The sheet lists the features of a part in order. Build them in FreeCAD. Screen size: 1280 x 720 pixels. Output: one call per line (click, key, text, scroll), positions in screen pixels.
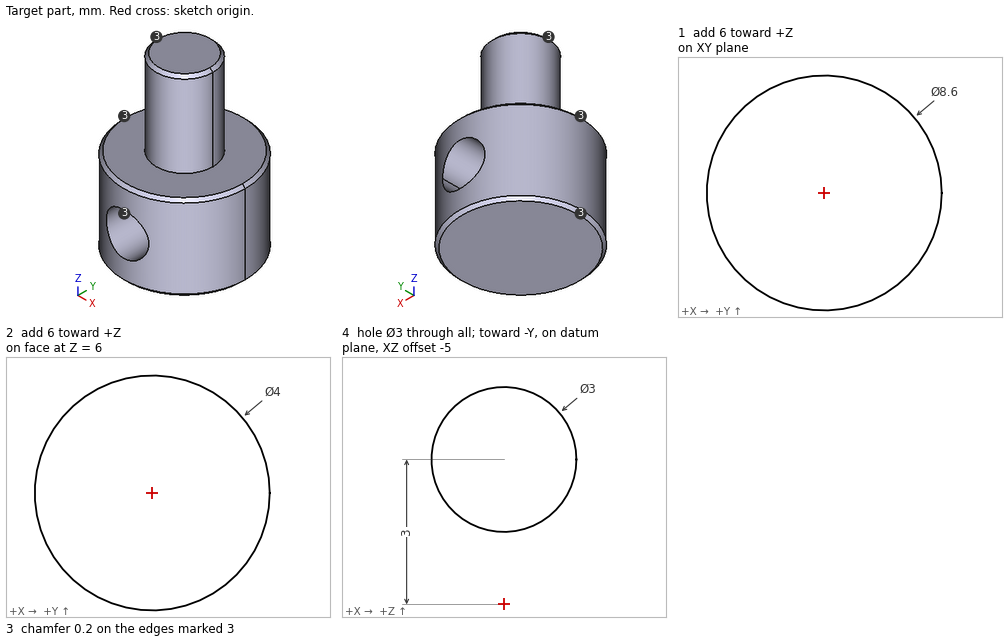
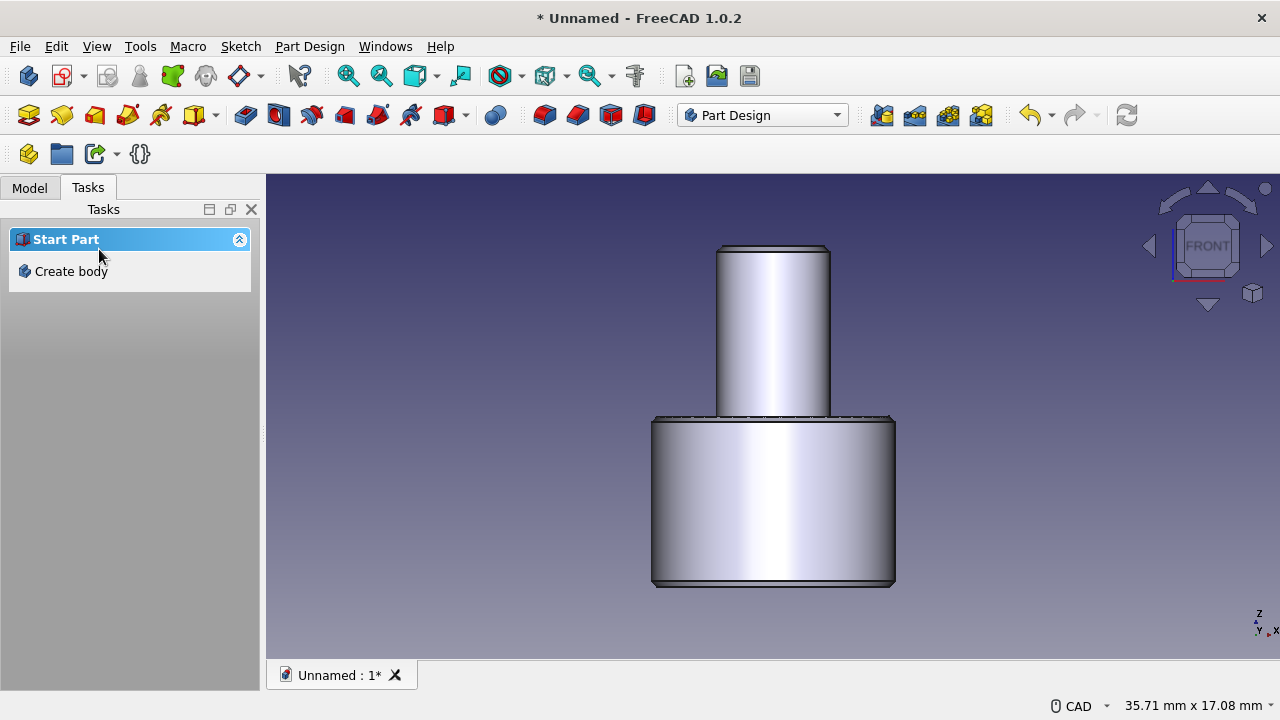
click(30, 188)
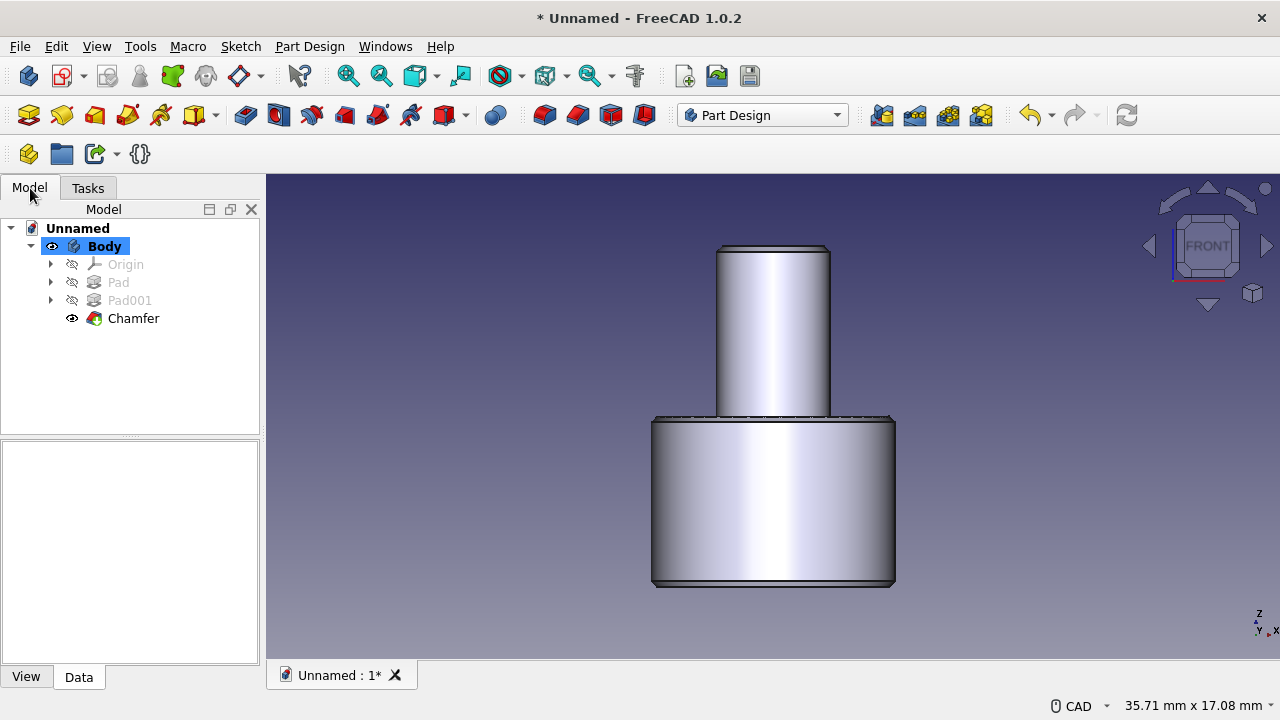
click(51, 264)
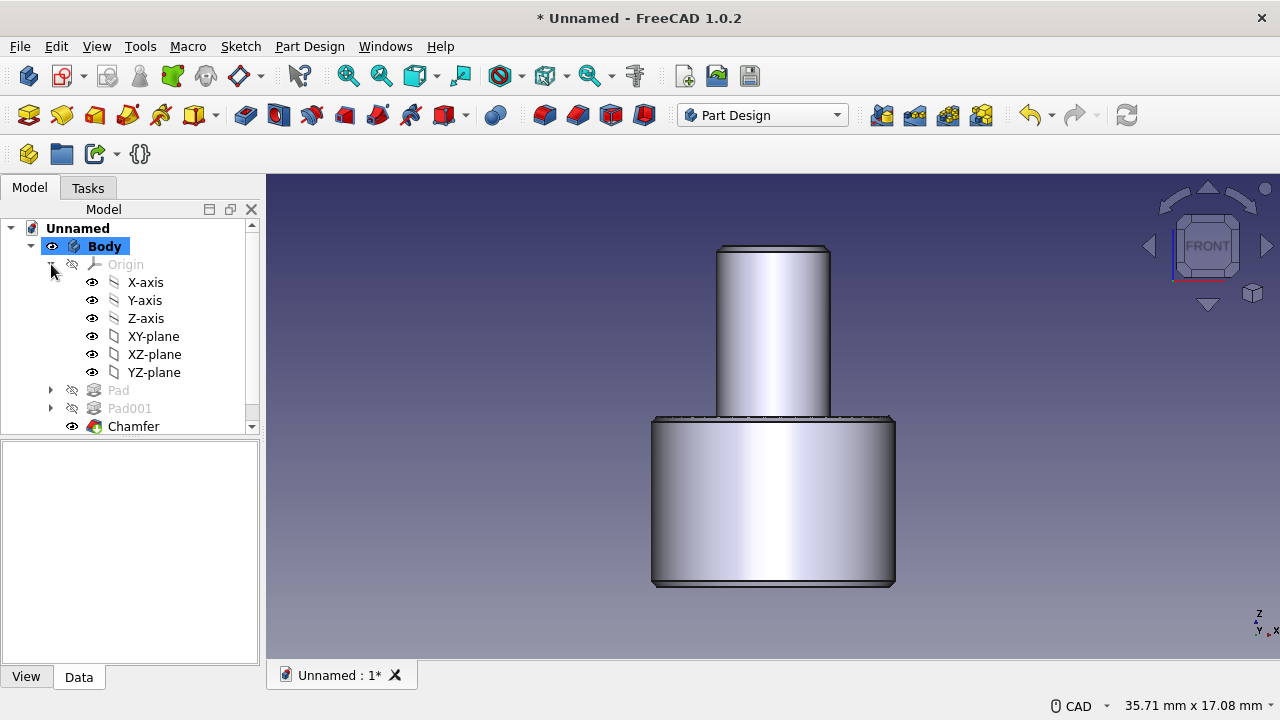
click(137, 354)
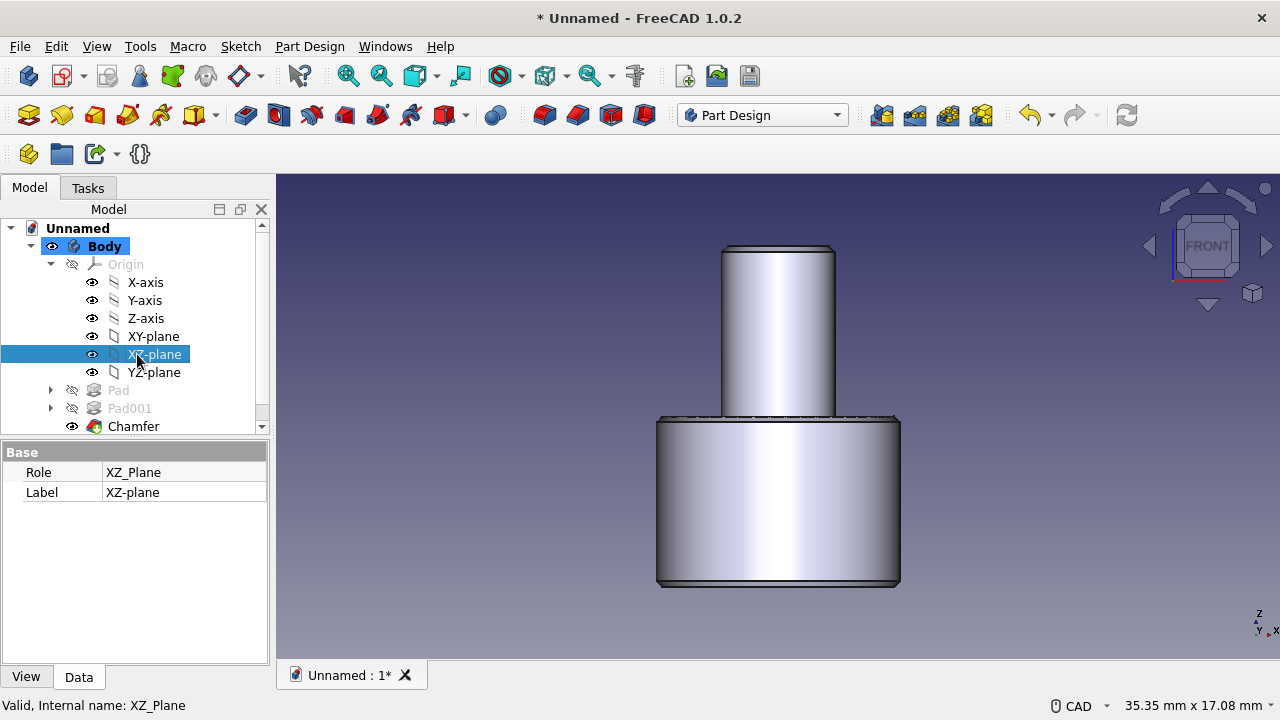
click(238, 76)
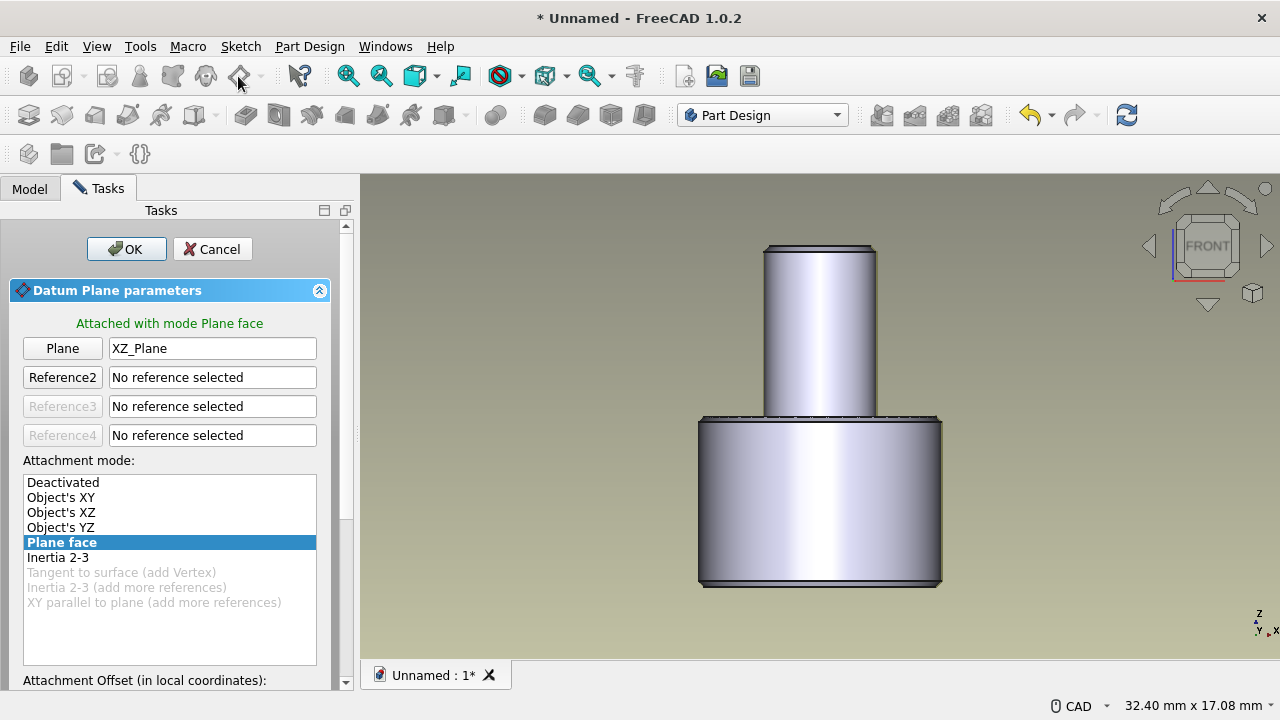
scroll(346, 455, down, 3)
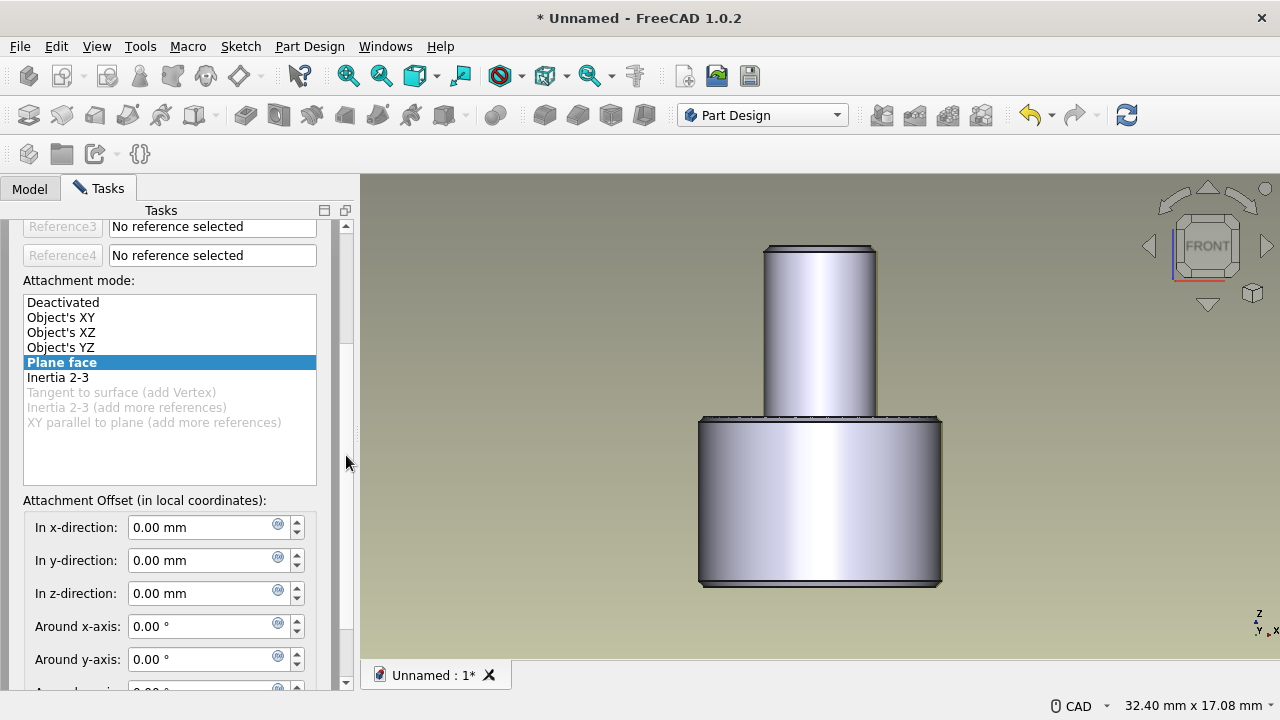
triple_click(210, 594)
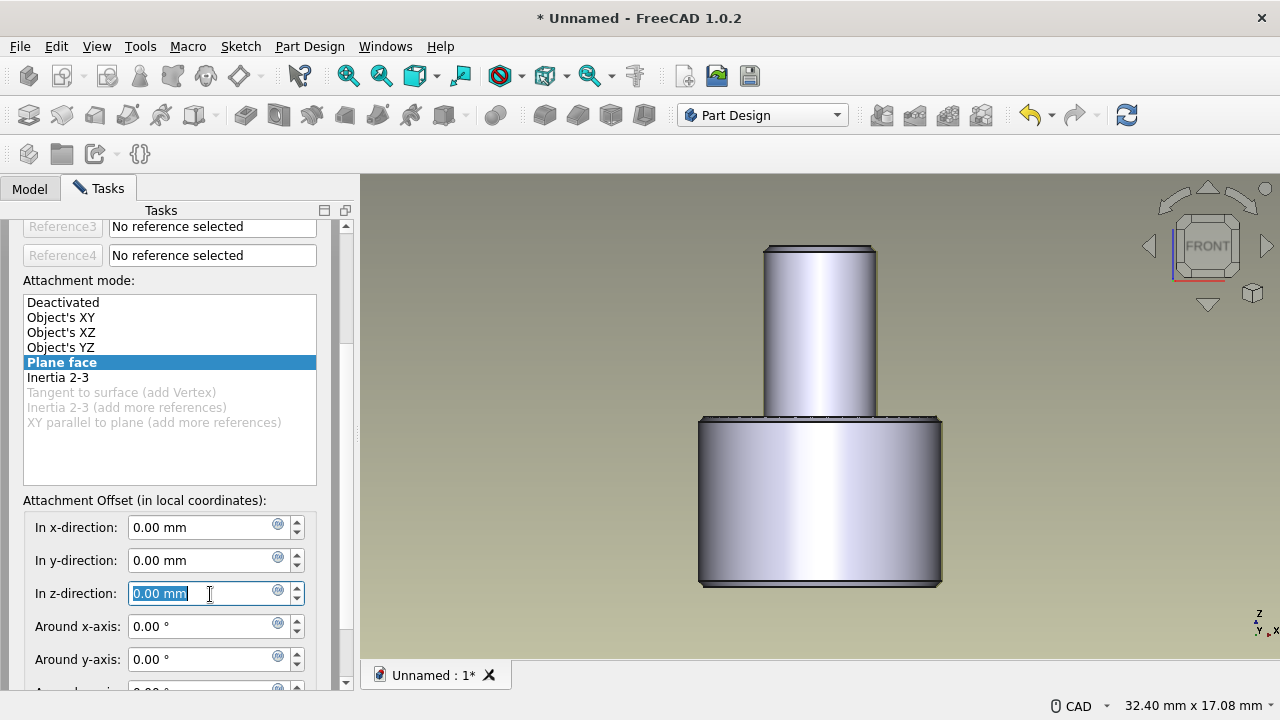
text(-5)
key(Tab)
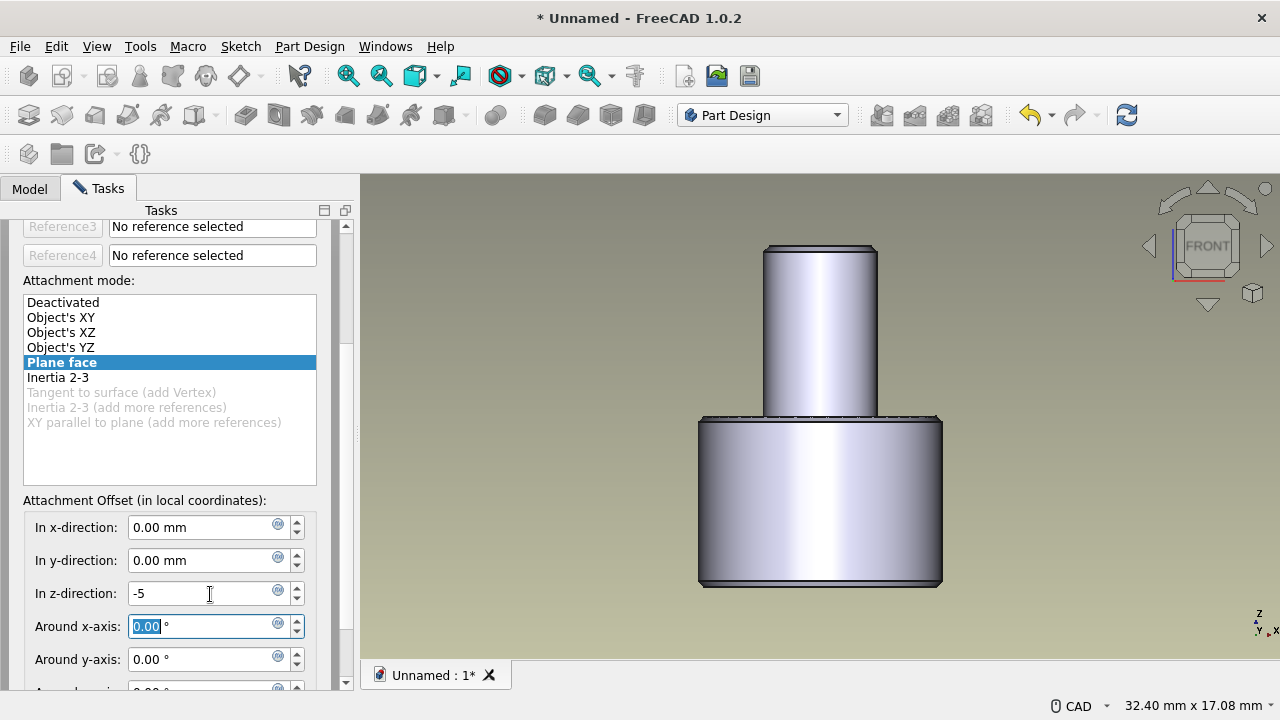
scroll(346, 455, up, 4)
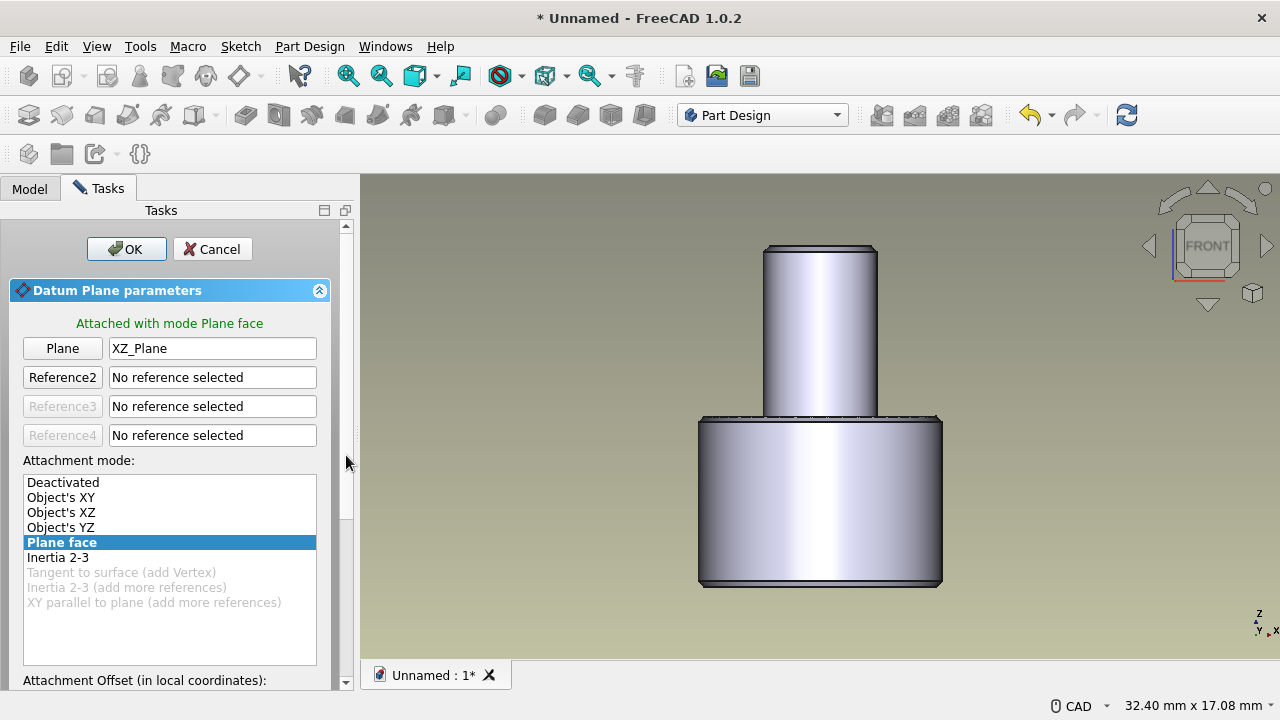
click(127, 249)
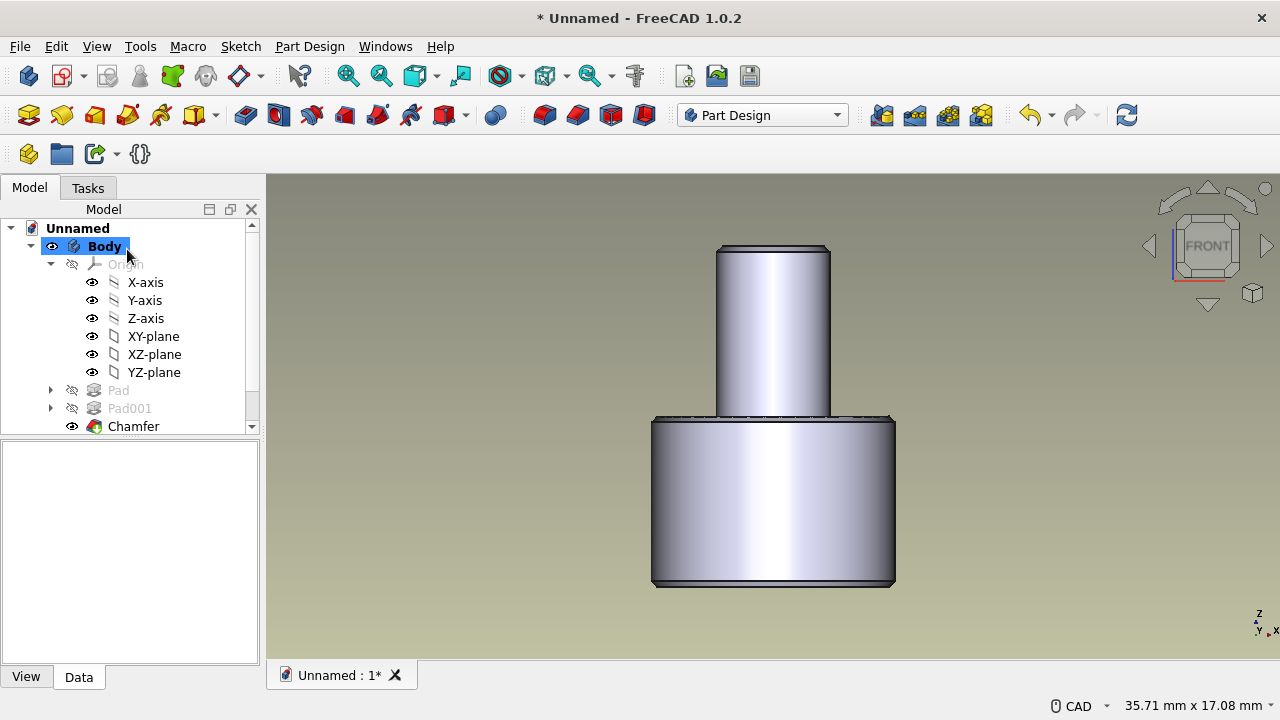
scroll(101, 332, down, 3)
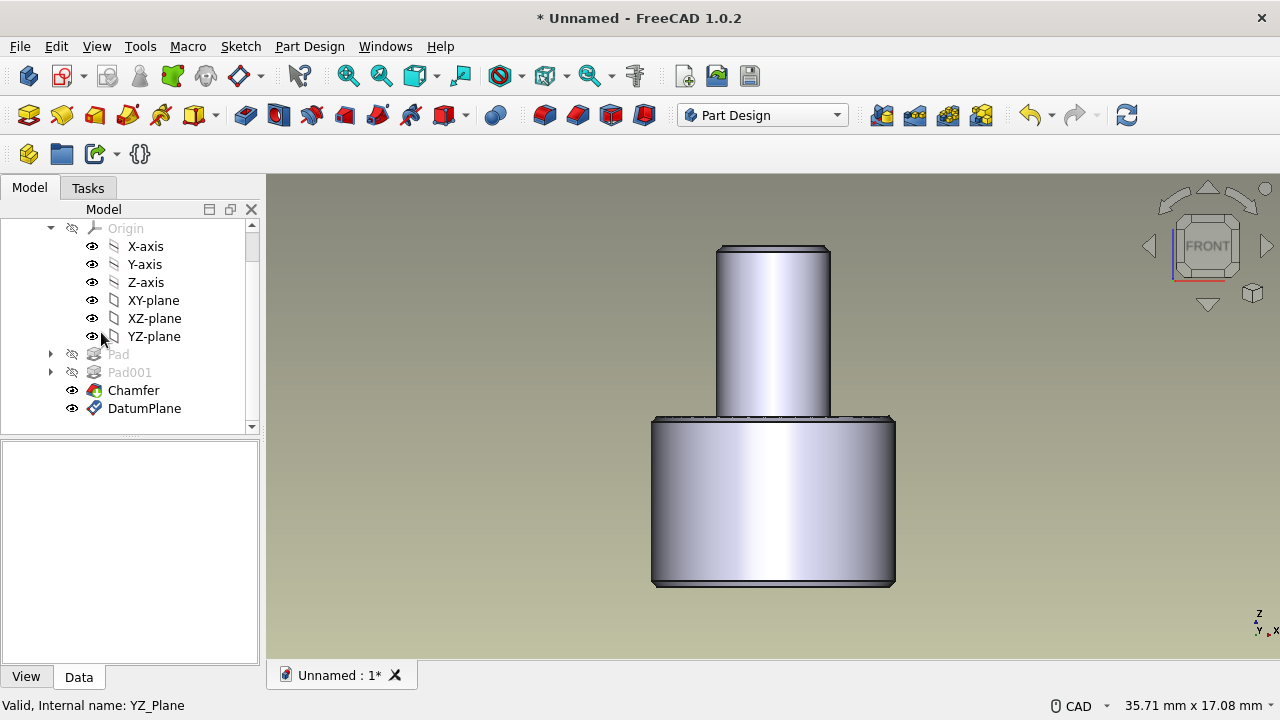
click(117, 408)